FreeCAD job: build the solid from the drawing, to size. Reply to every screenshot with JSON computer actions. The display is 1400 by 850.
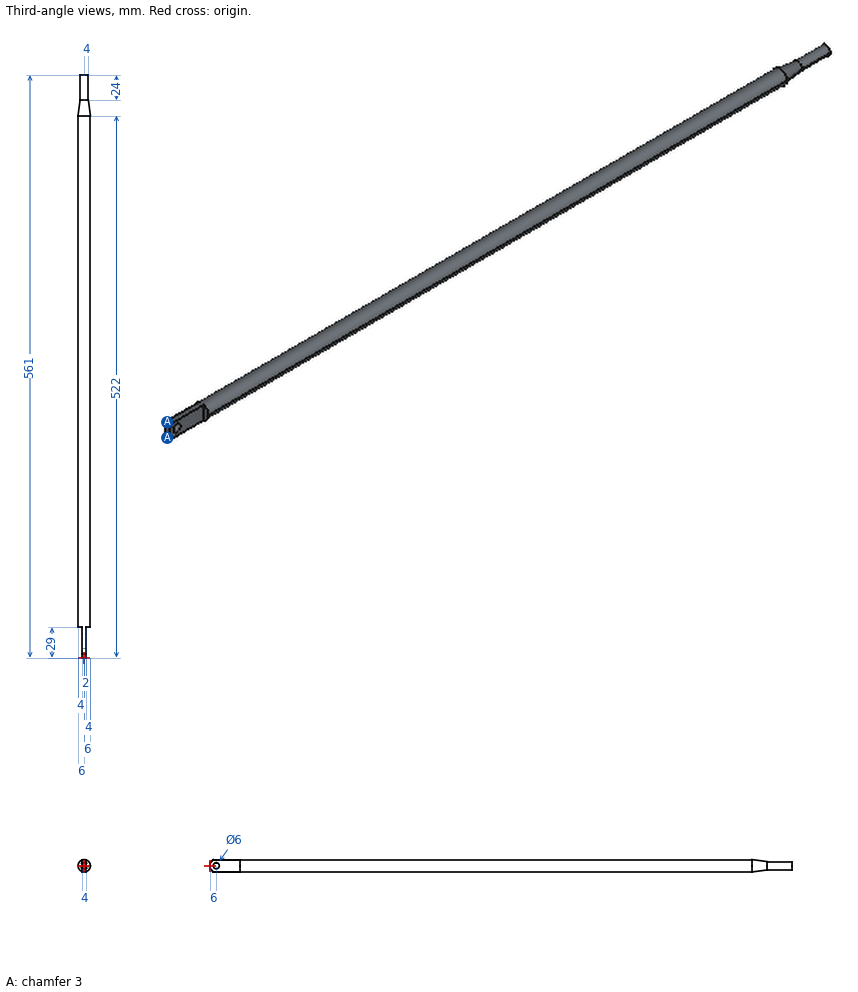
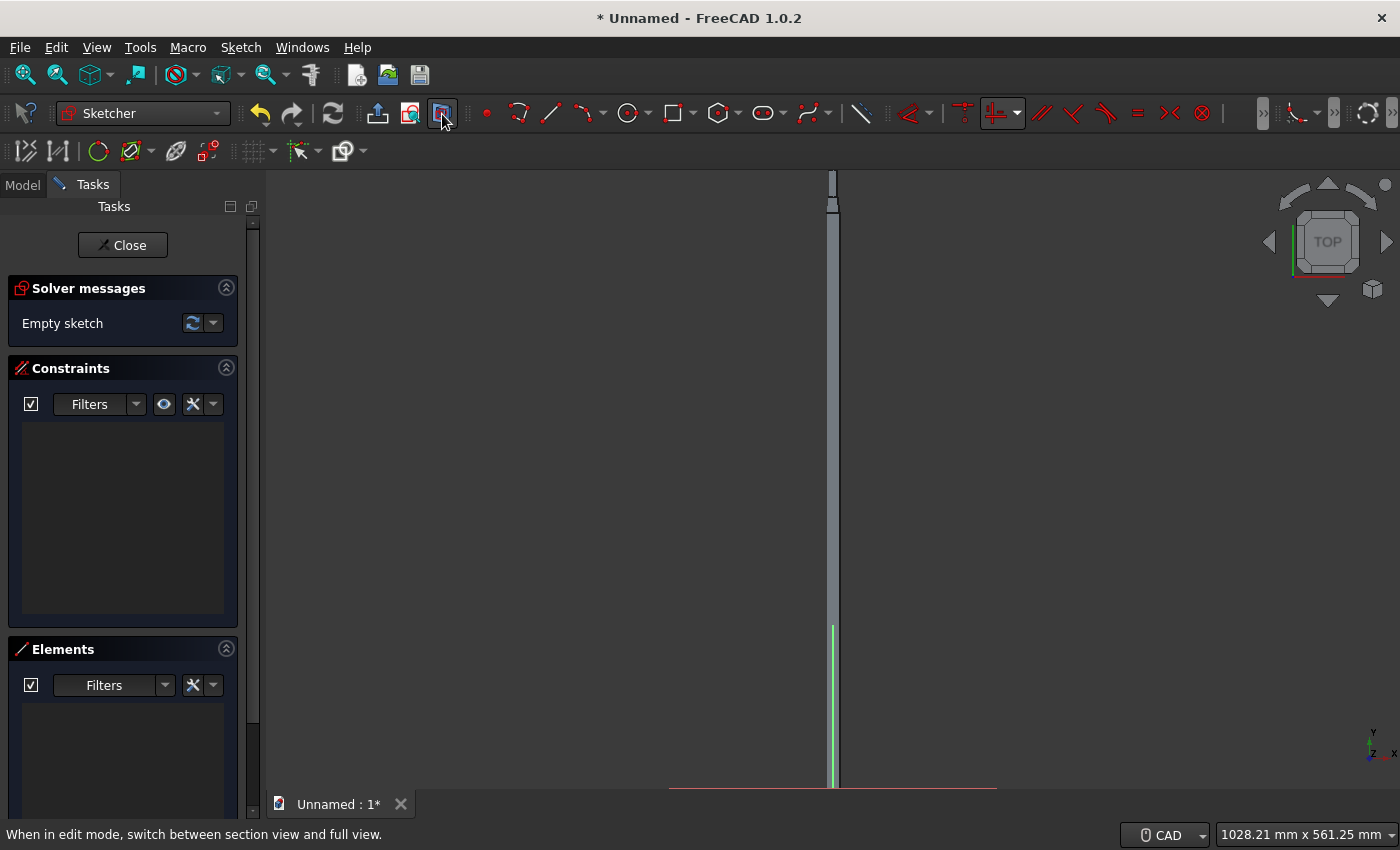
{"action": "scroll", "coordinate": [764, 480], "scroll_direction": "down", "scroll_amount": 5}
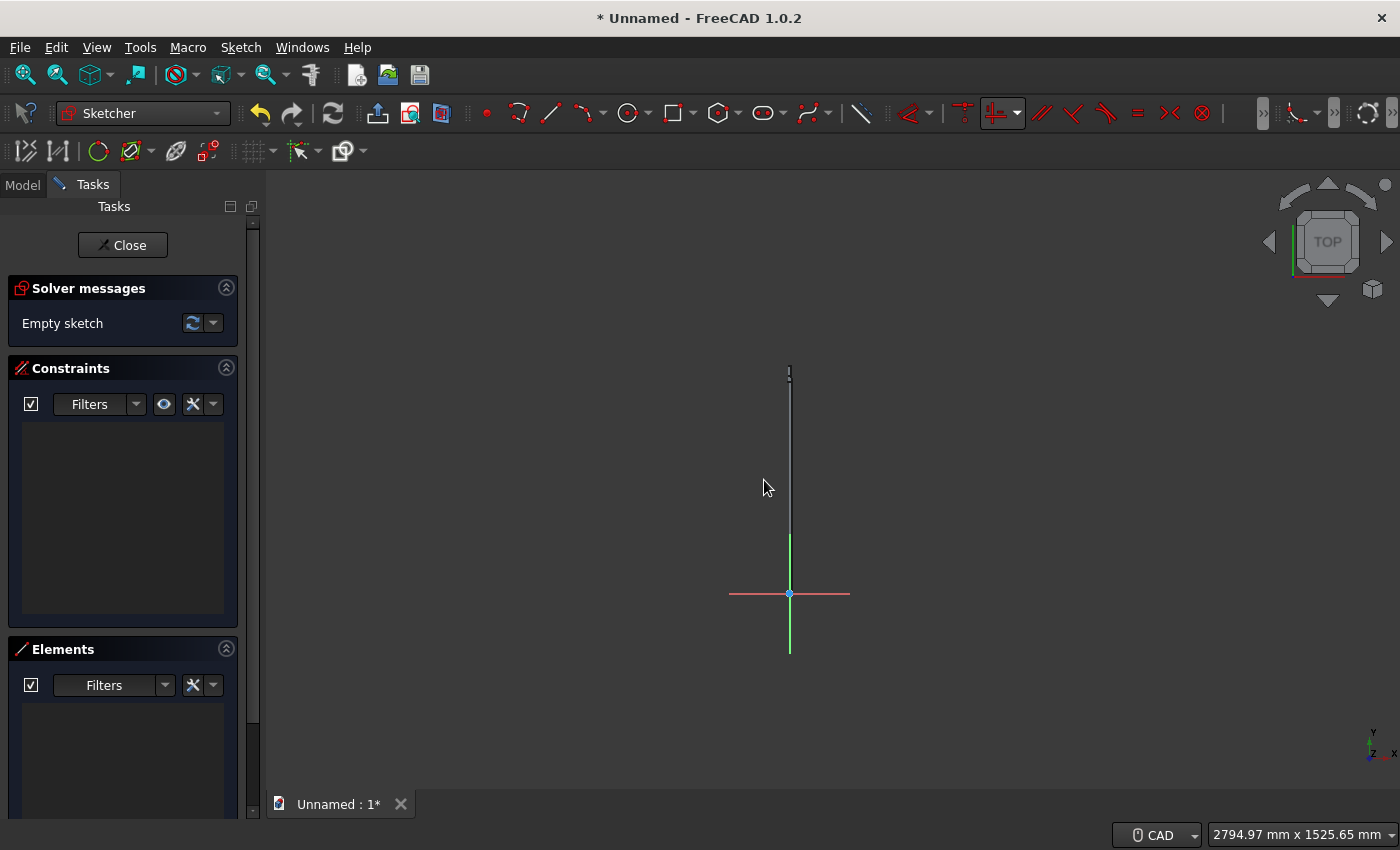
{"action": "scroll", "coordinate": [790, 594], "scroll_direction": "up", "scroll_amount": 15}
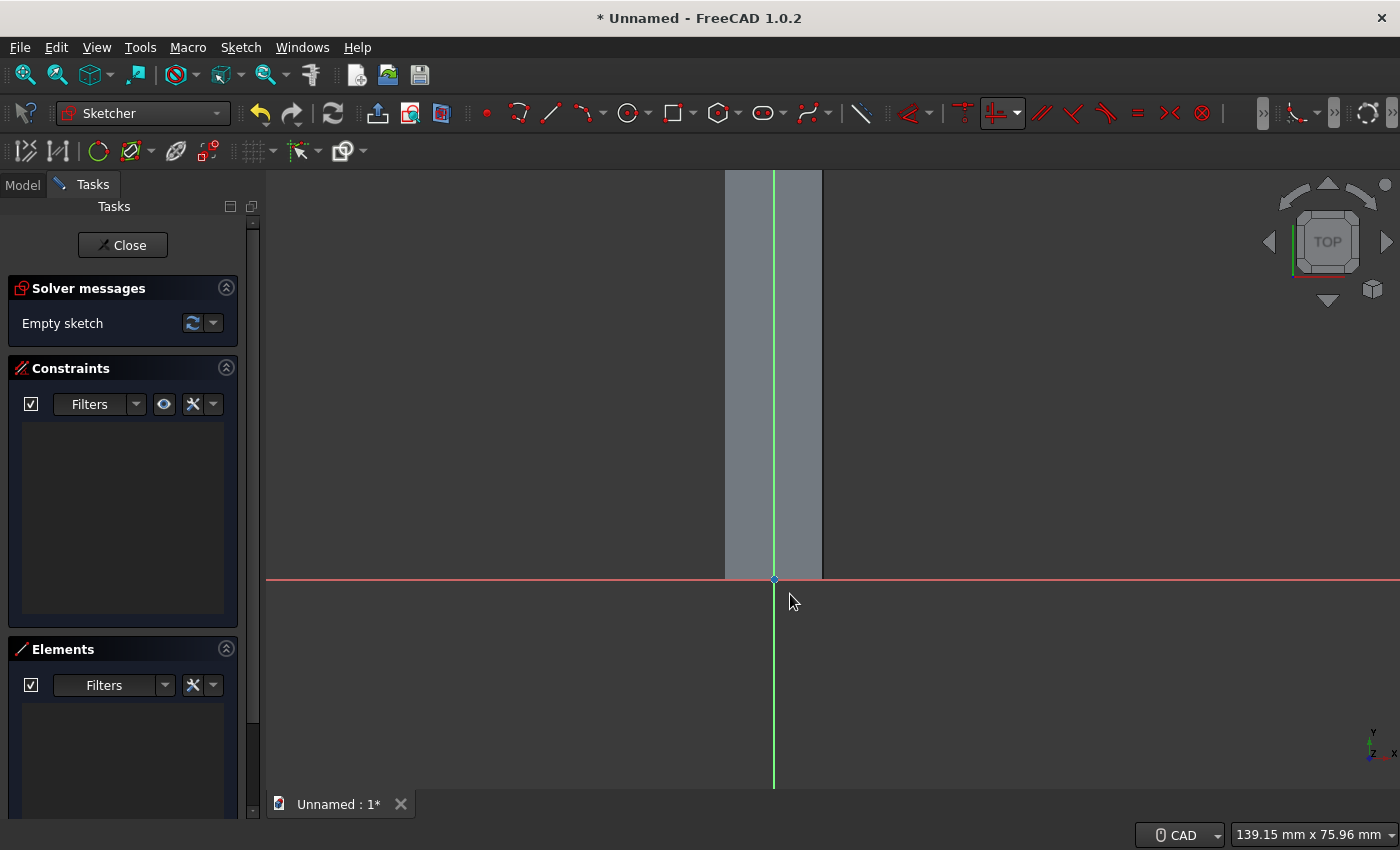
{"action": "scroll", "coordinate": [732, 440], "scroll_direction": "up", "scroll_amount": 3}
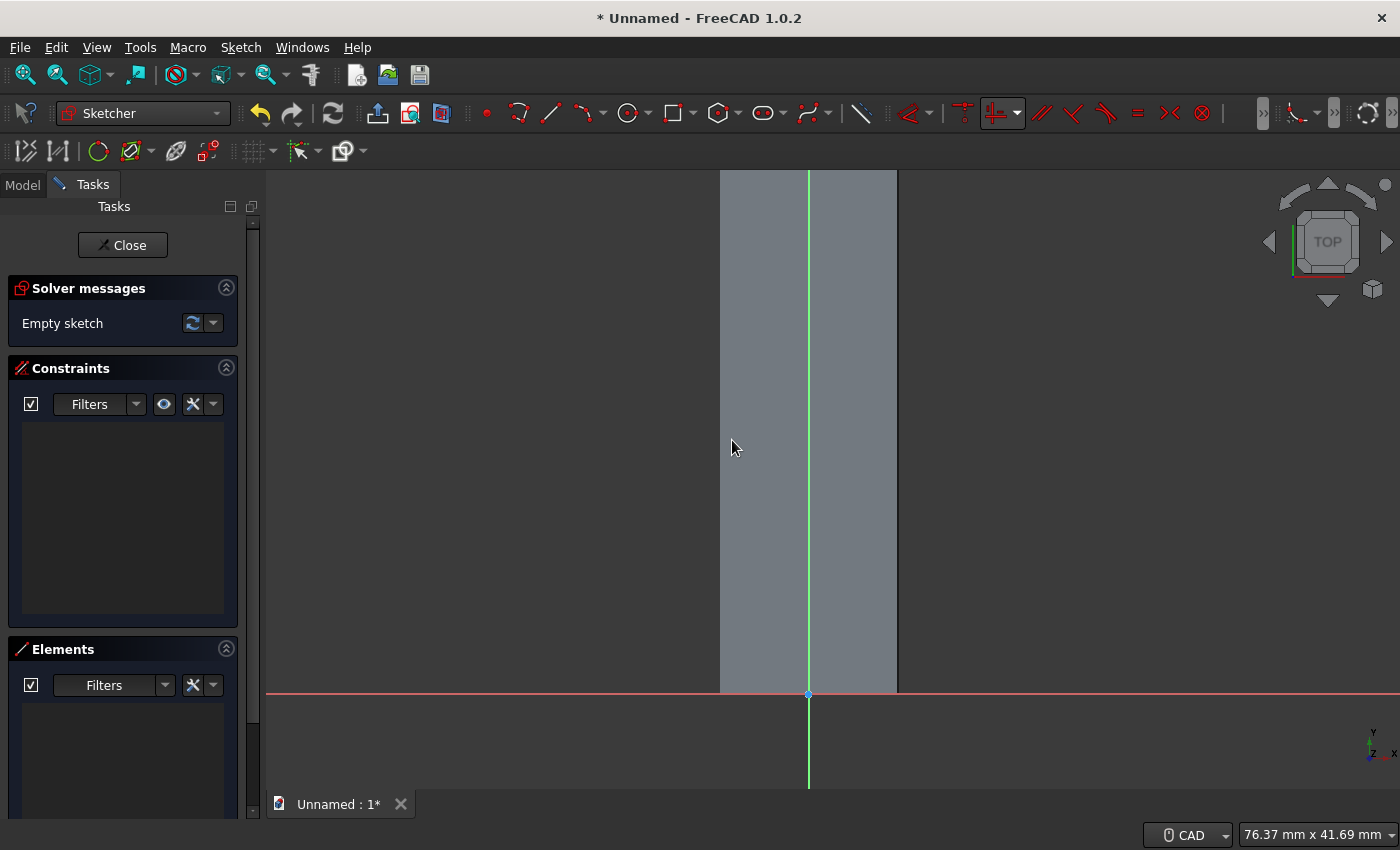
{"action": "left_click", "coordinate": [674, 114]}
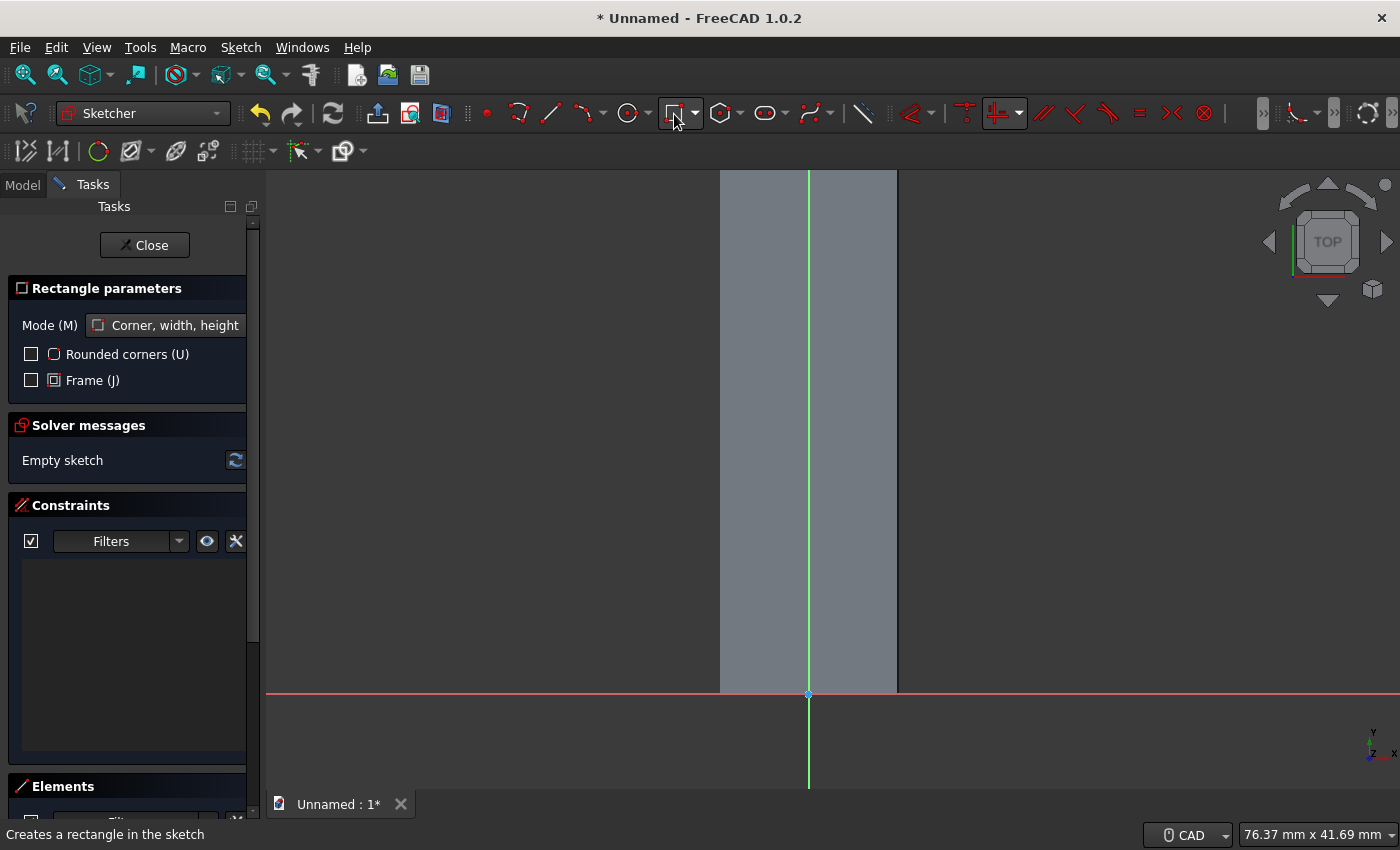
{"action": "left_click", "coordinate": [720, 264]}
{"action": "left_click", "coordinate": [779, 694]}
{"action": "key", "text": "Escape"}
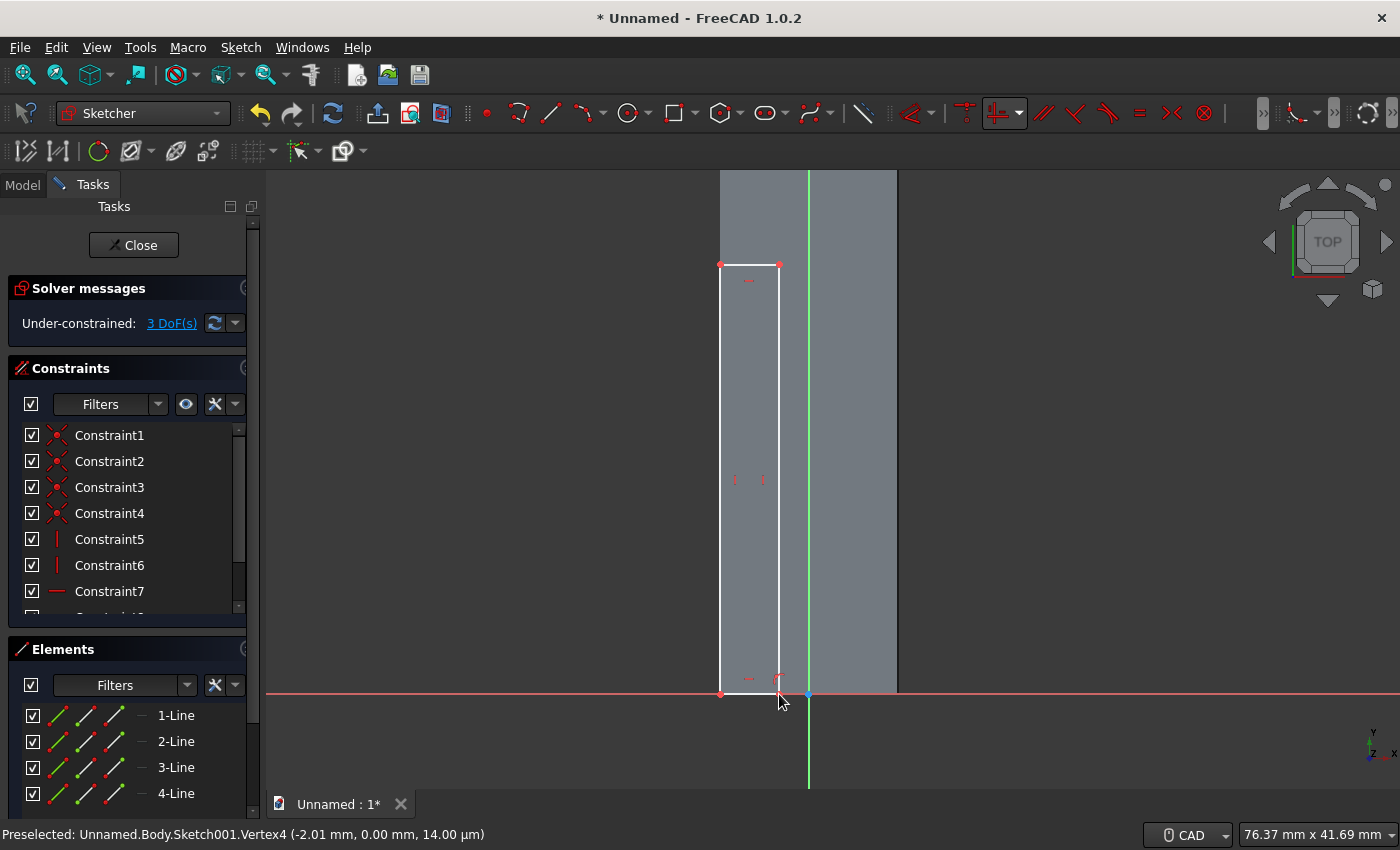
{"action": "left_click", "coordinate": [910, 114]}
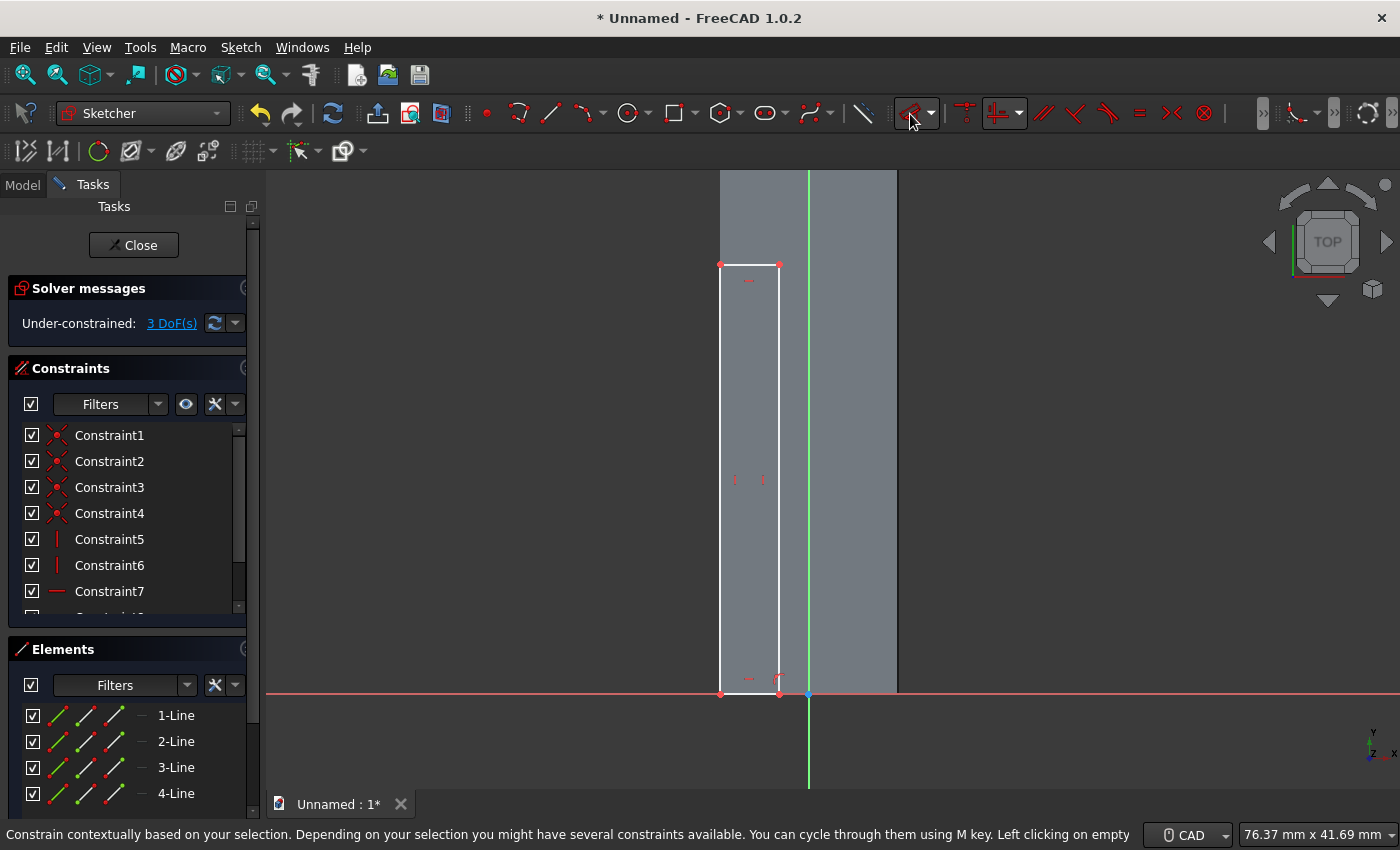
{"action": "left_click", "coordinate": [738, 694]}
{"action": "left_click", "coordinate": [750, 728]}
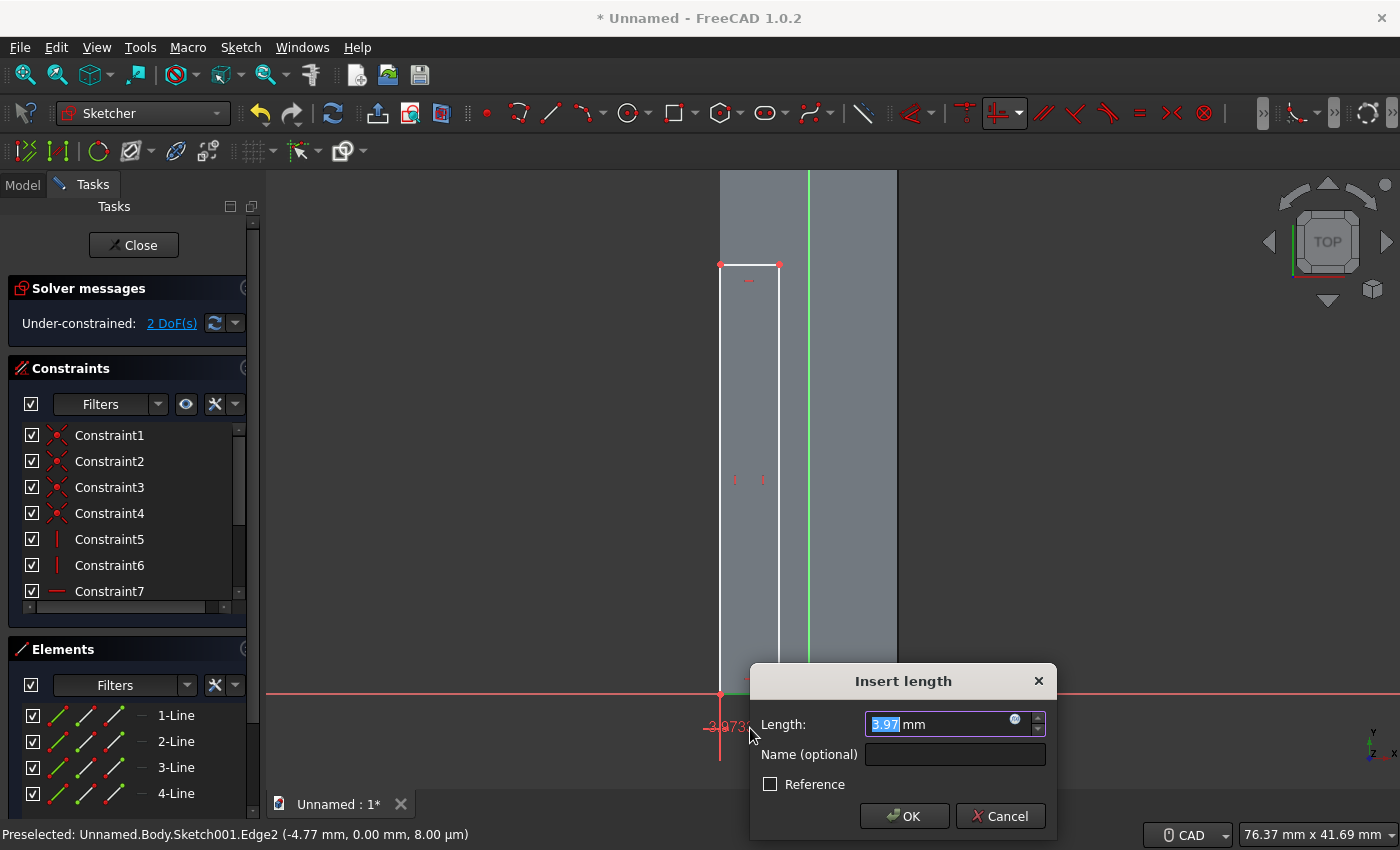
{"action": "type", "text": "4"}
{"action": "key", "text": "Return"}